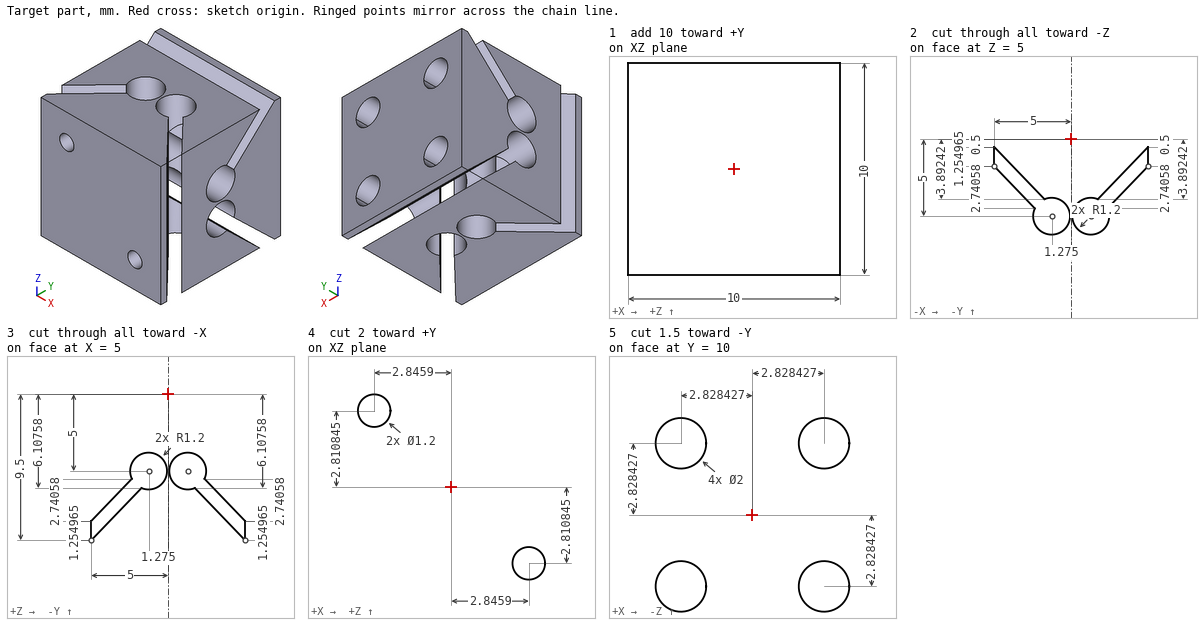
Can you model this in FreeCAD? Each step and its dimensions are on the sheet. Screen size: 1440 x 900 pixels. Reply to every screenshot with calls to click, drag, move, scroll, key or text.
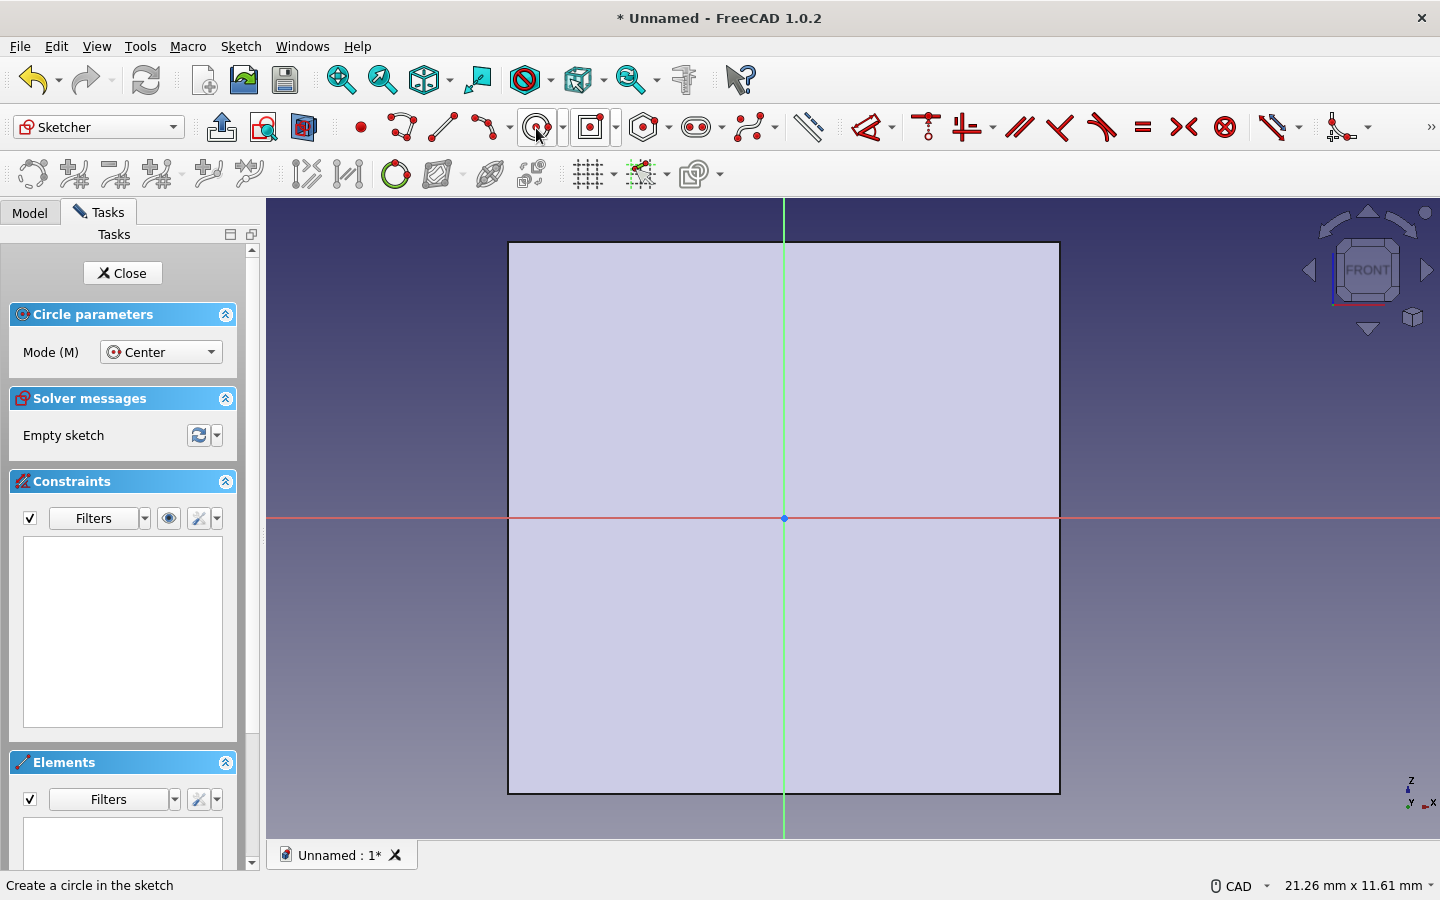
click(627, 363)
move(651, 339)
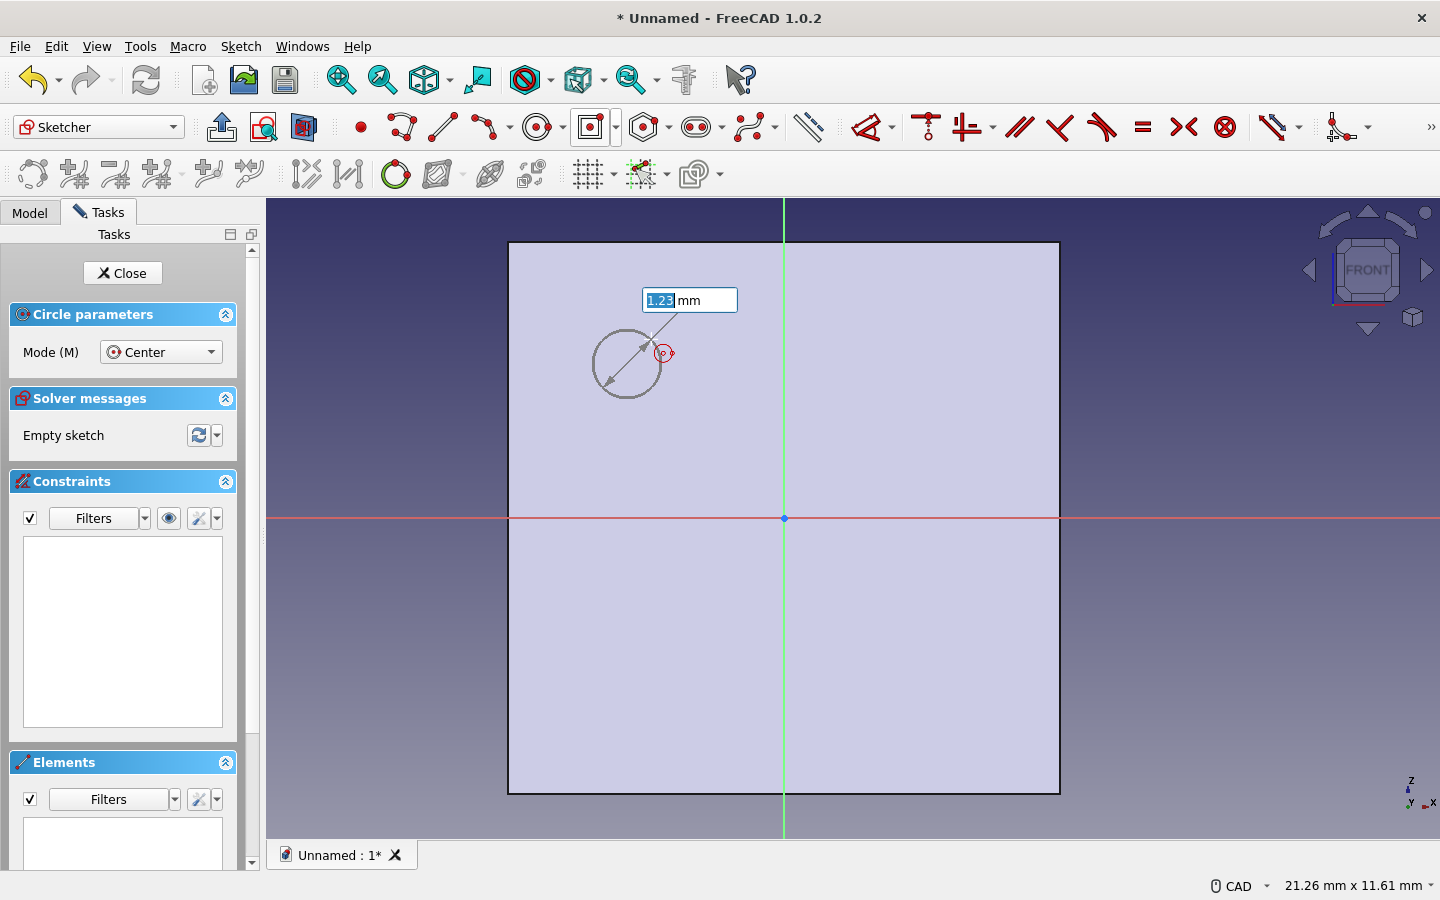
text(1.2)
key(Return)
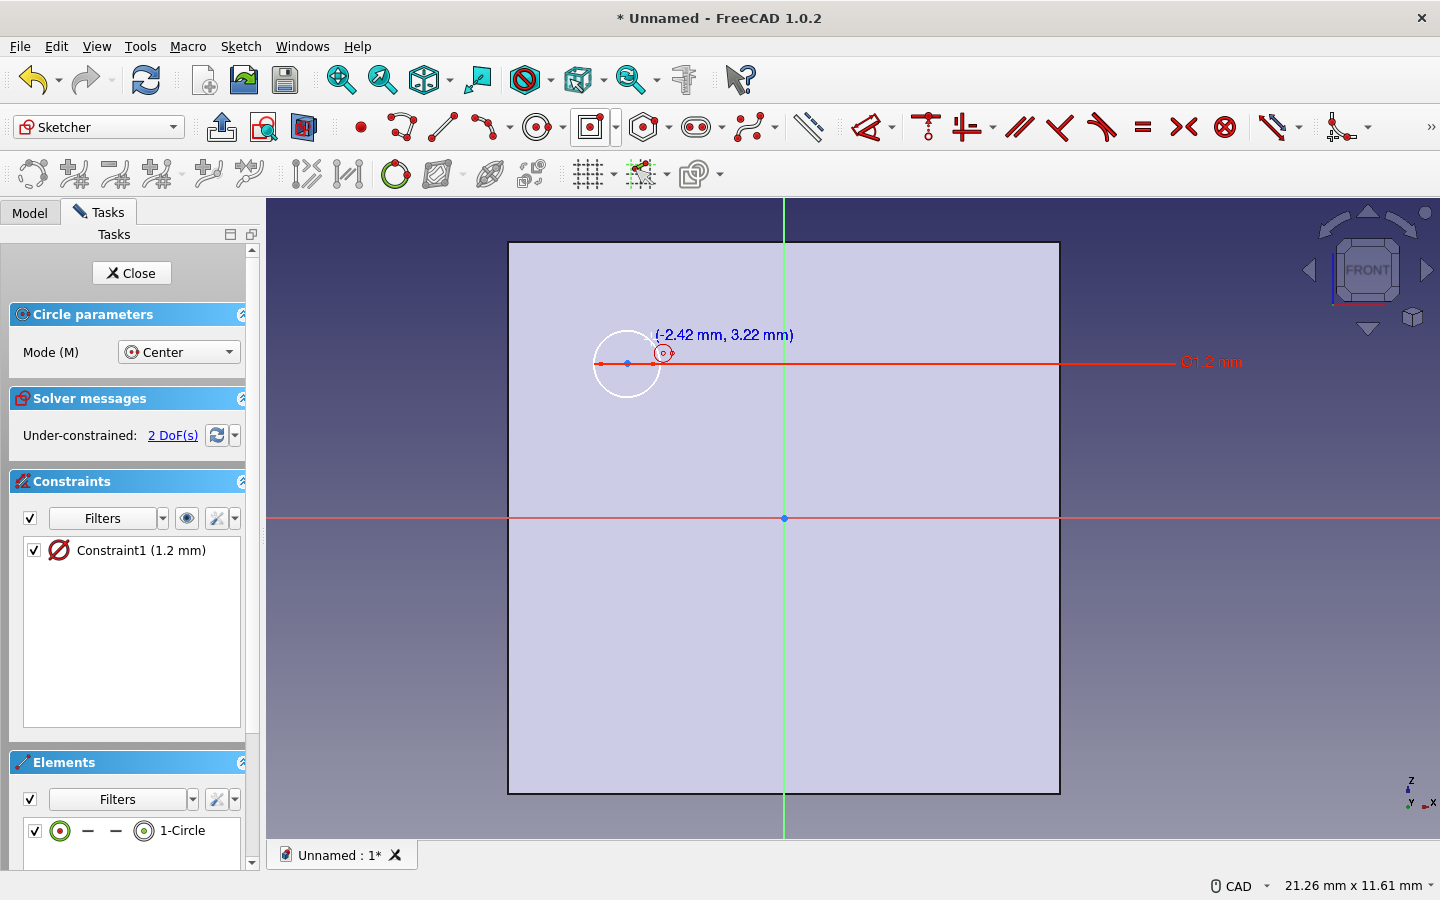
click(941, 673)
move(965, 650)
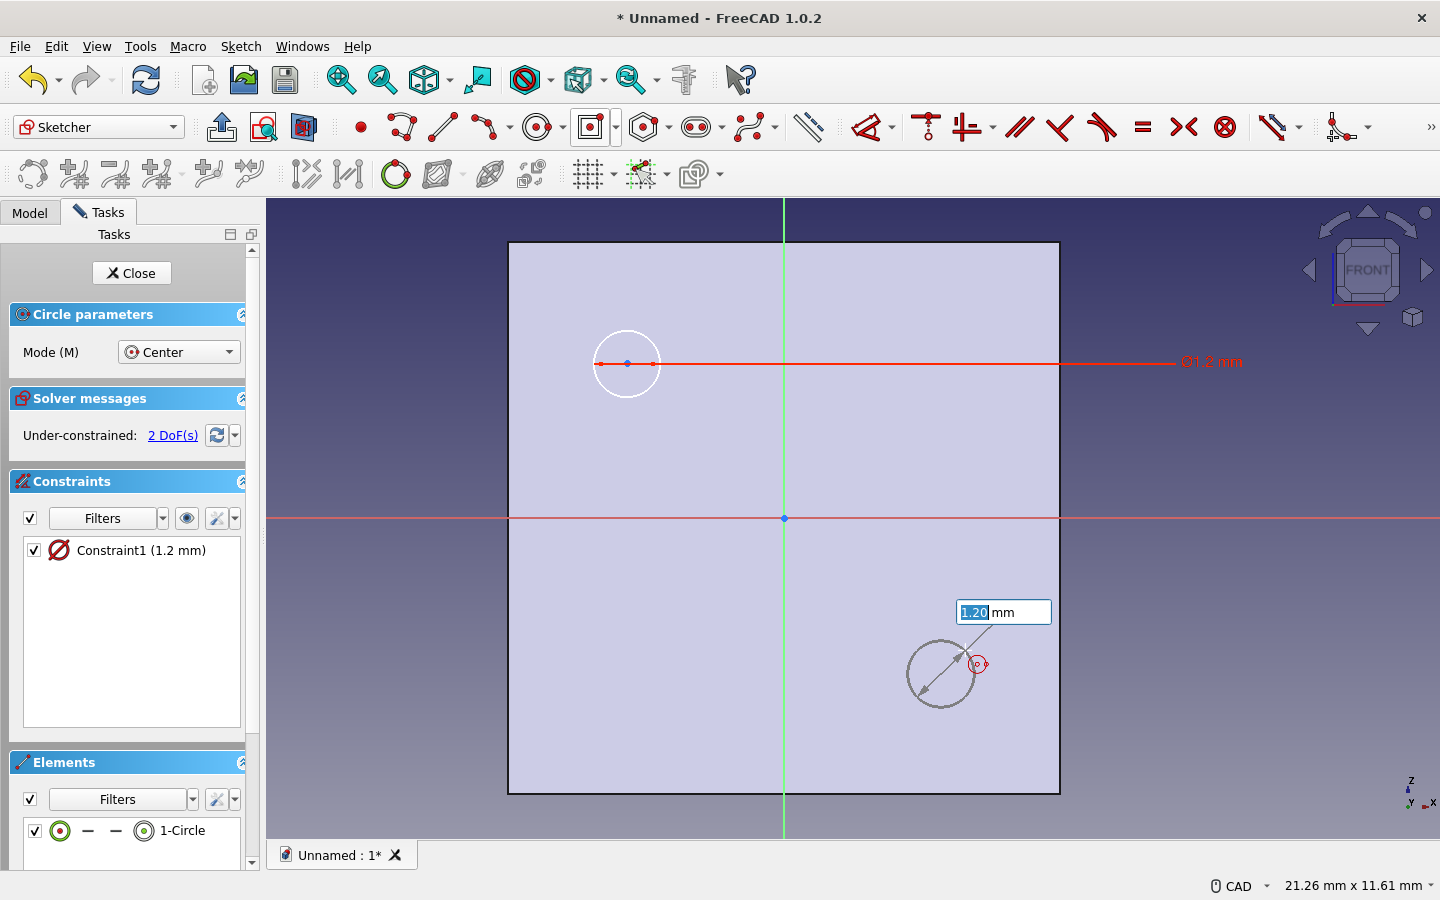
text(1.2)
key(Return)
key(Escape)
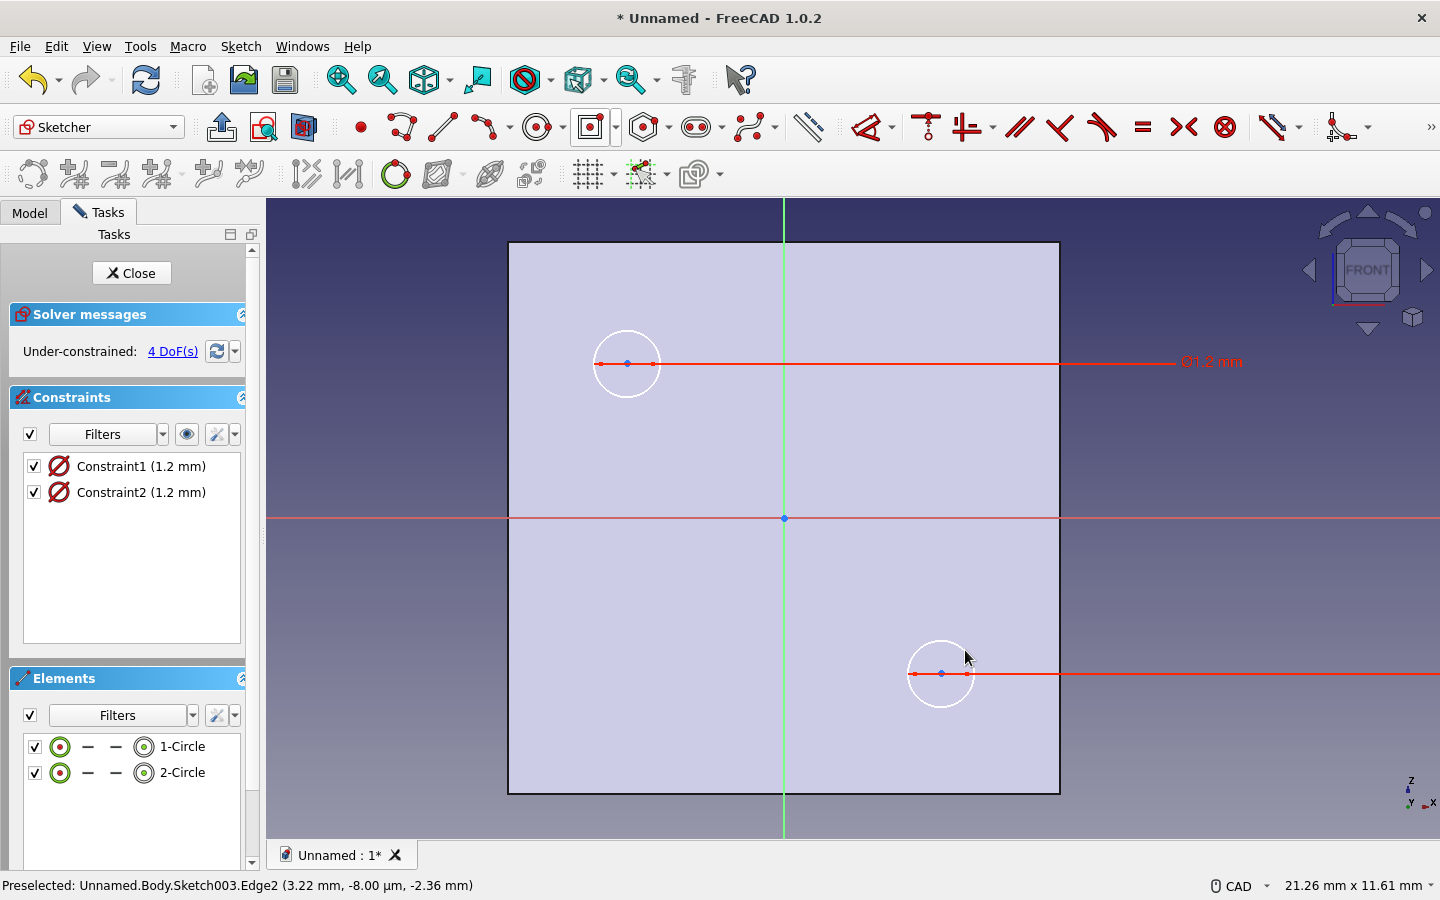
click(866, 128)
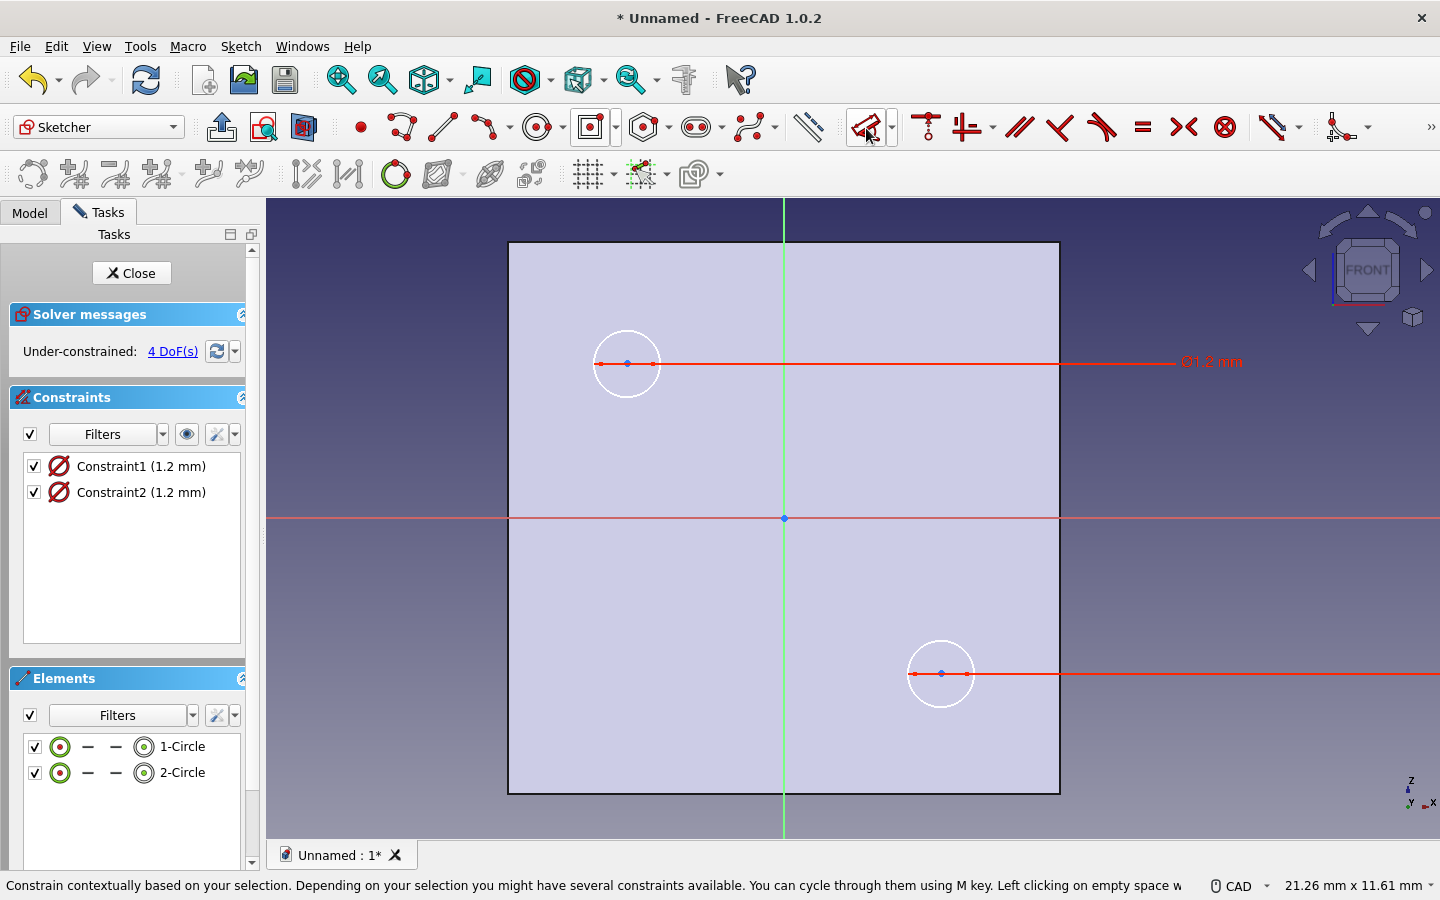
click(627, 364)
click(706, 330)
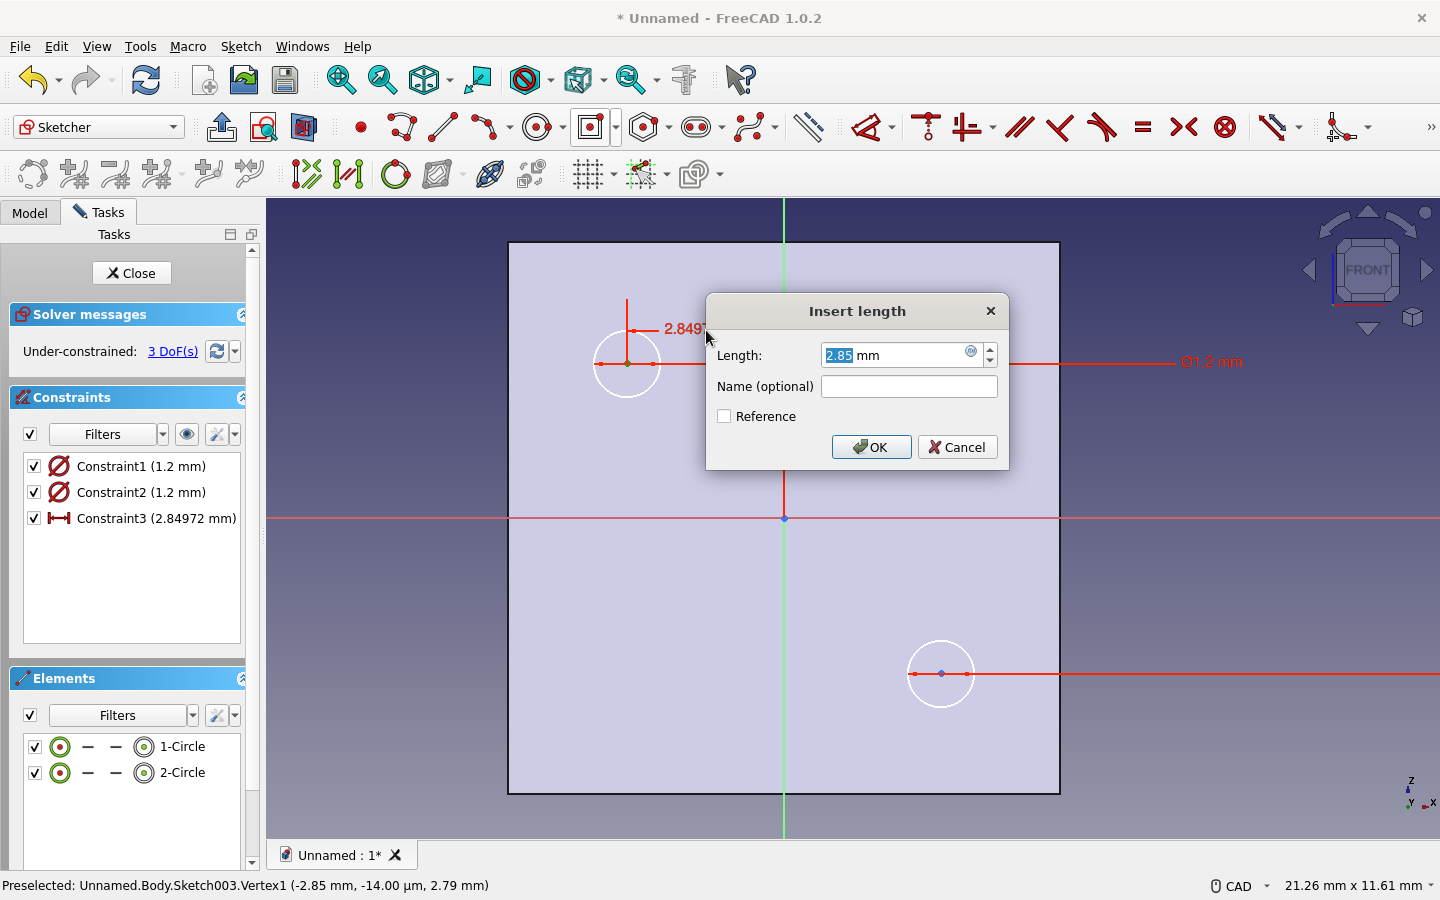
text(2.8459)
key(Return)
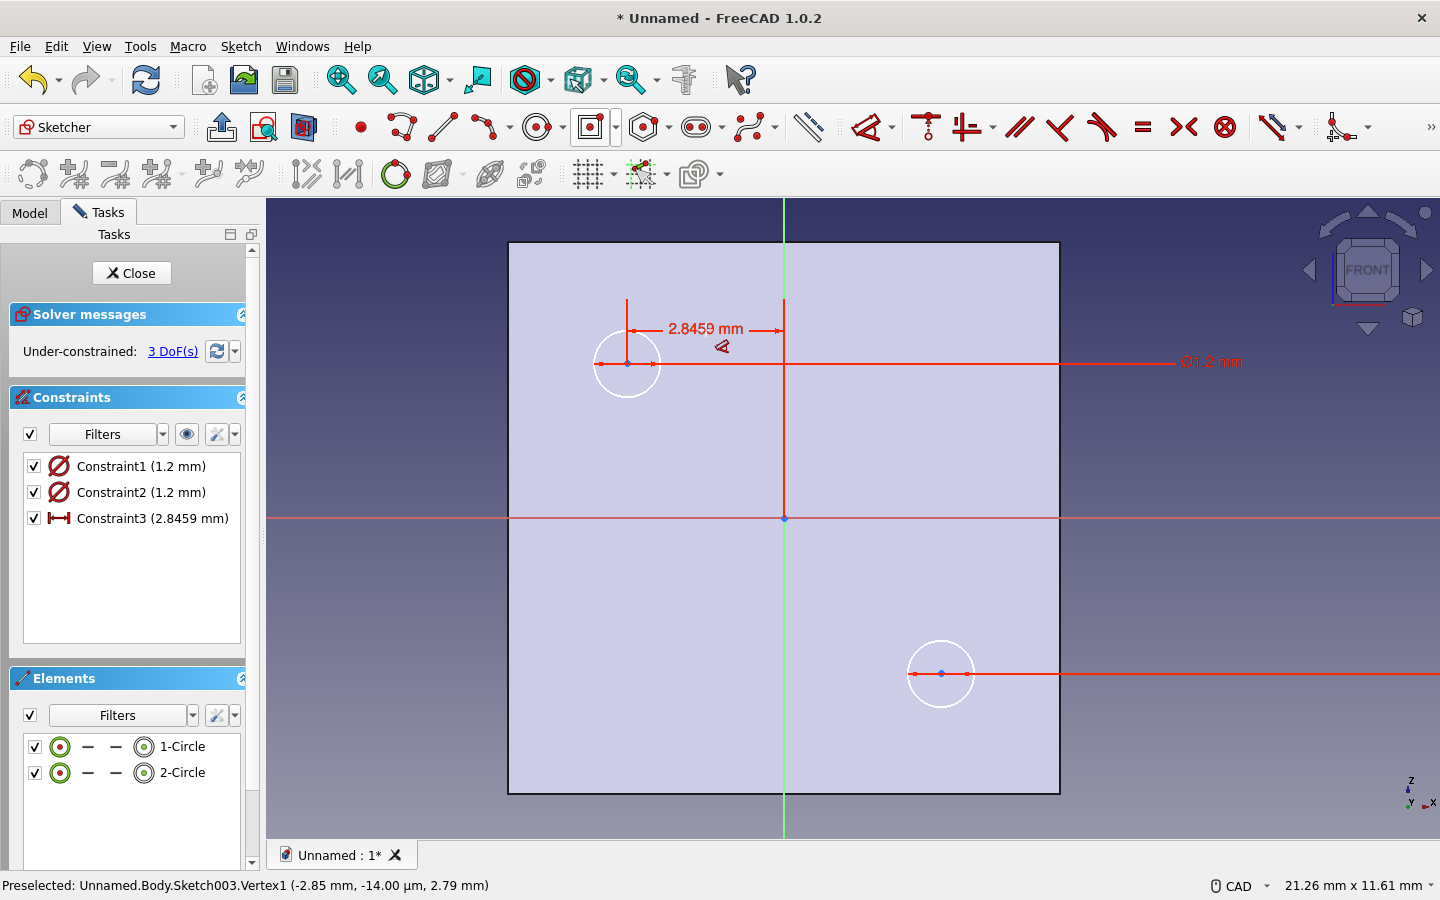
click(941, 674)
click(863, 708)